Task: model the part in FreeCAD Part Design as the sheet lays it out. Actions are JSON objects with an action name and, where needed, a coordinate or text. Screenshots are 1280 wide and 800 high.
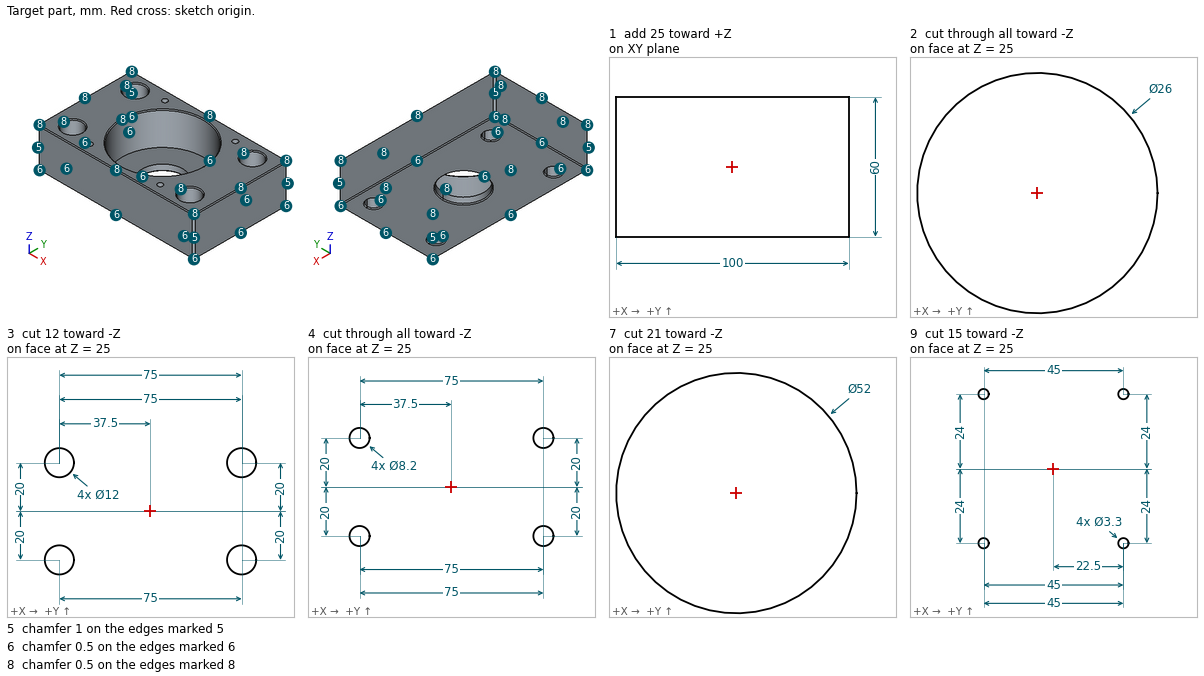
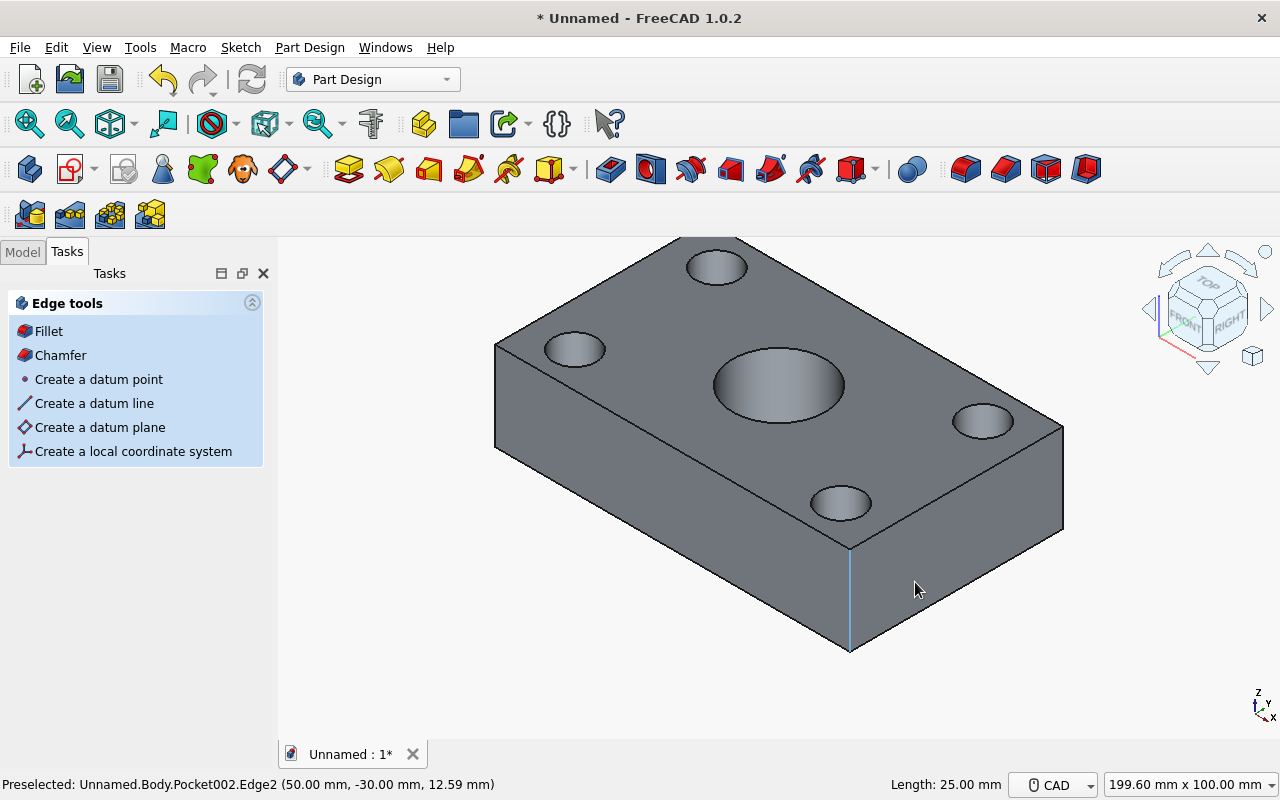
{"action": "key", "text": "v f"}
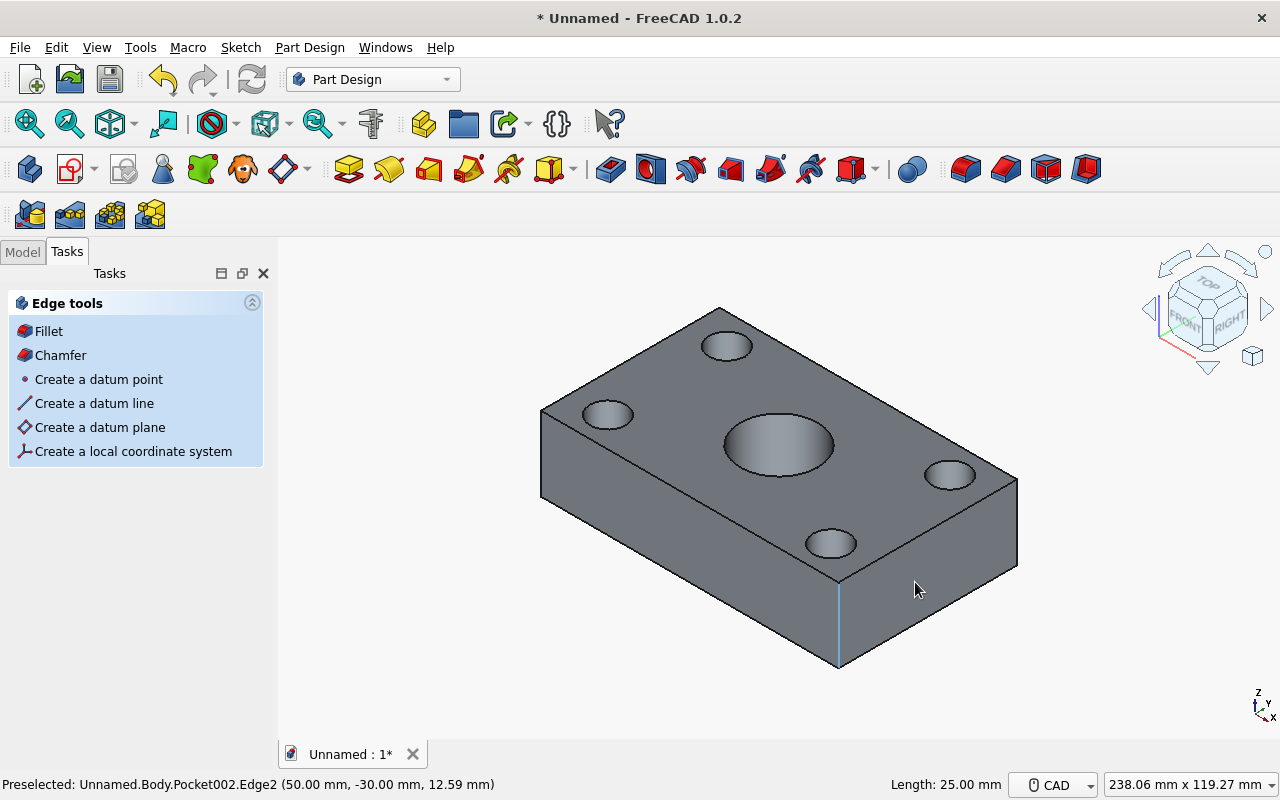
{"action": "key", "text": "2"}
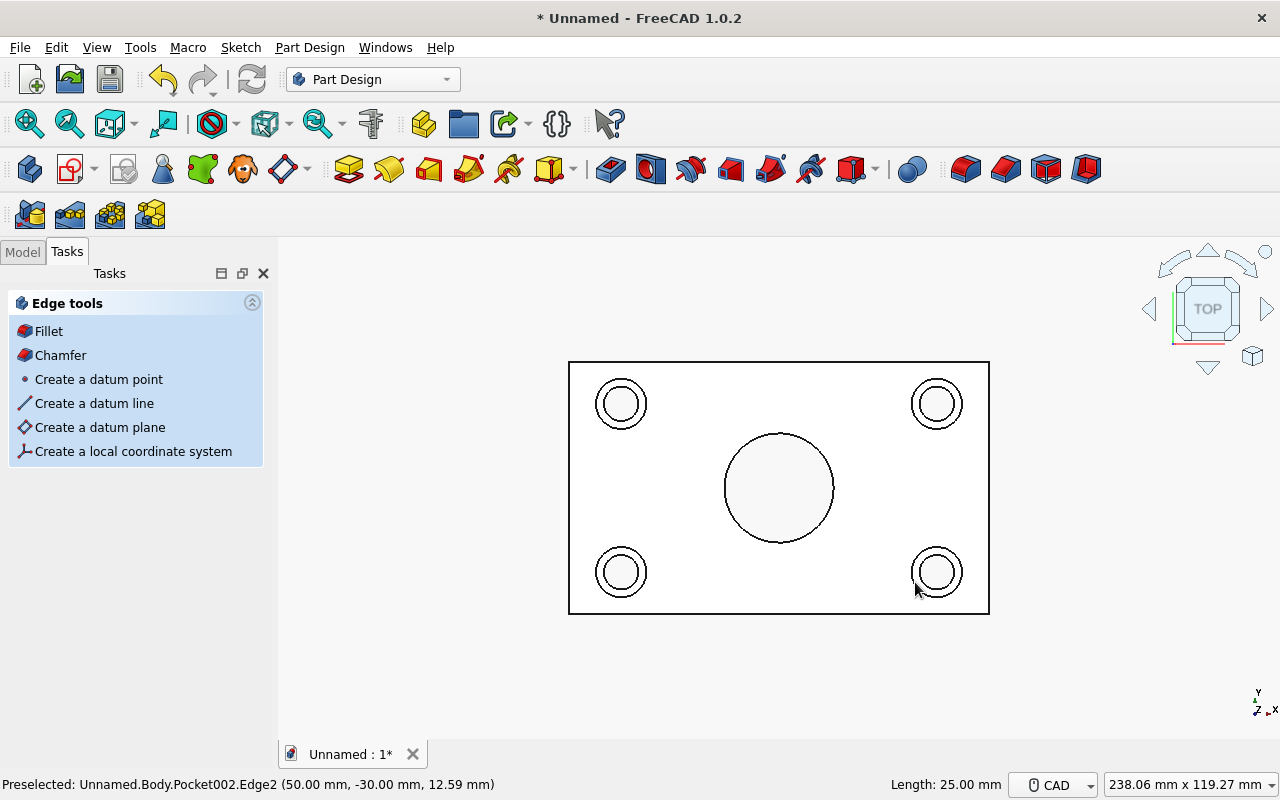
{"action": "key", "text": "1"}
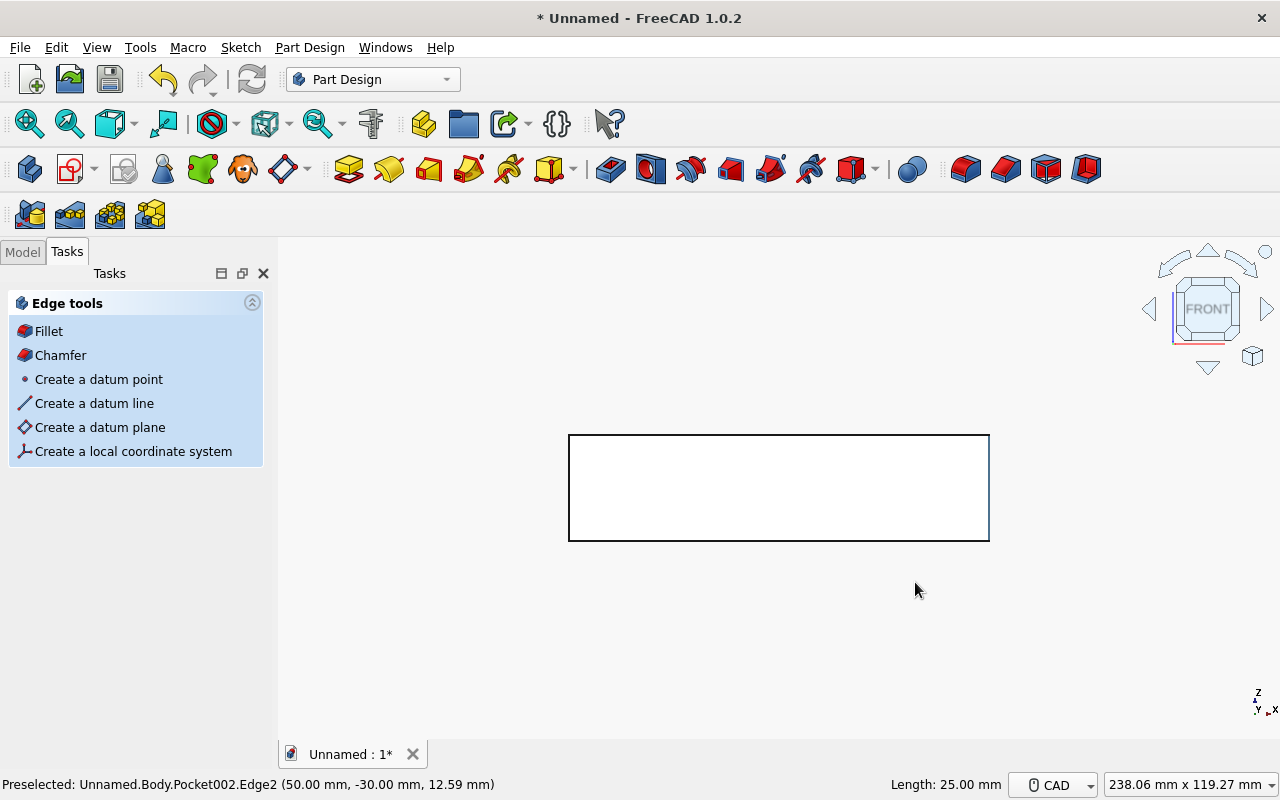
{"action": "left_click", "coordinate": [30, 124]}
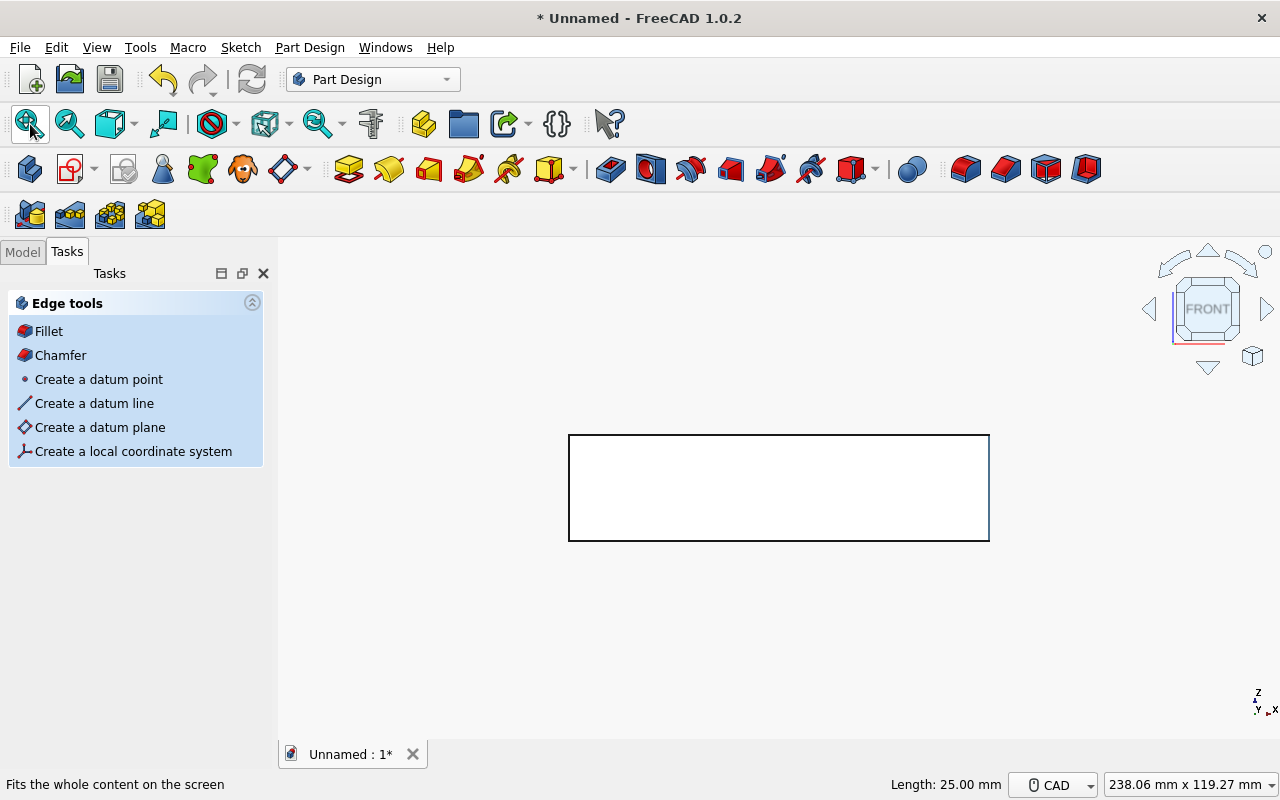
{"action": "left_click", "coordinate": [569, 487], "text": "ctrl"}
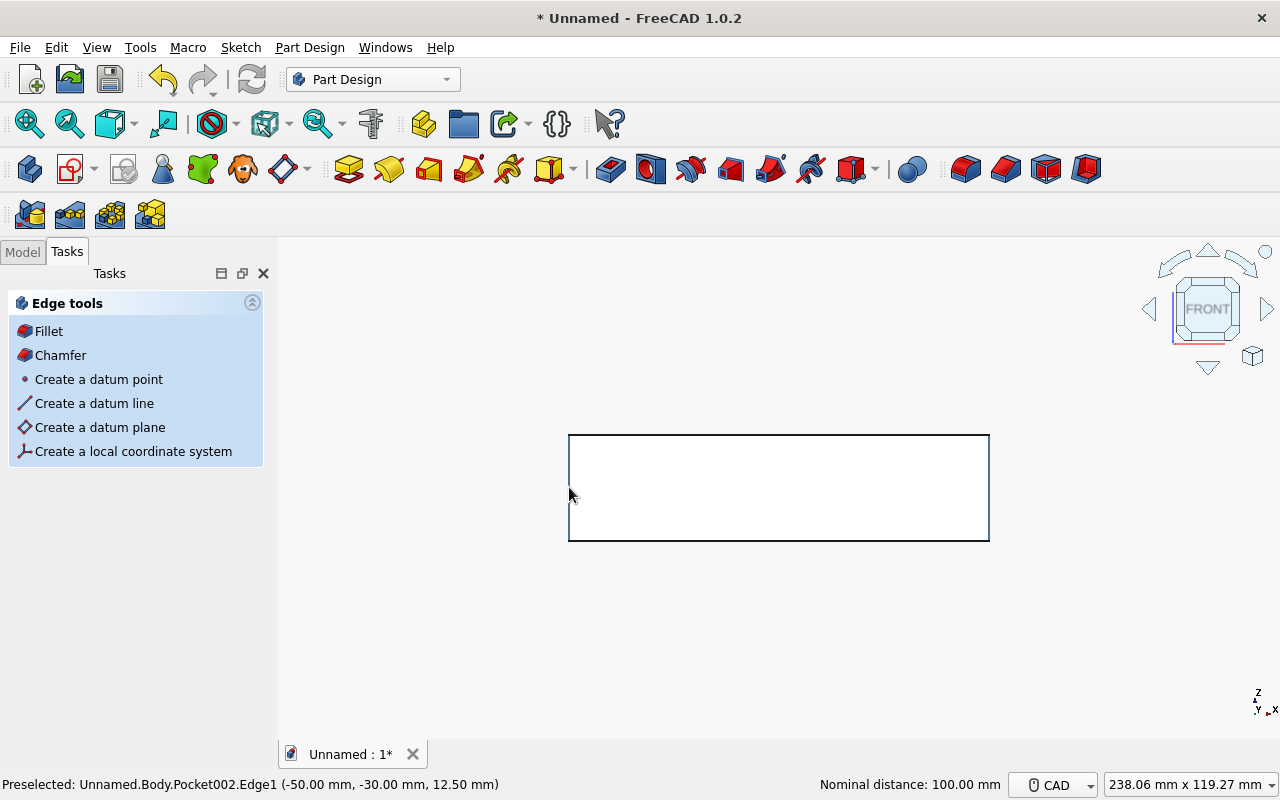
{"action": "key", "text": "3"}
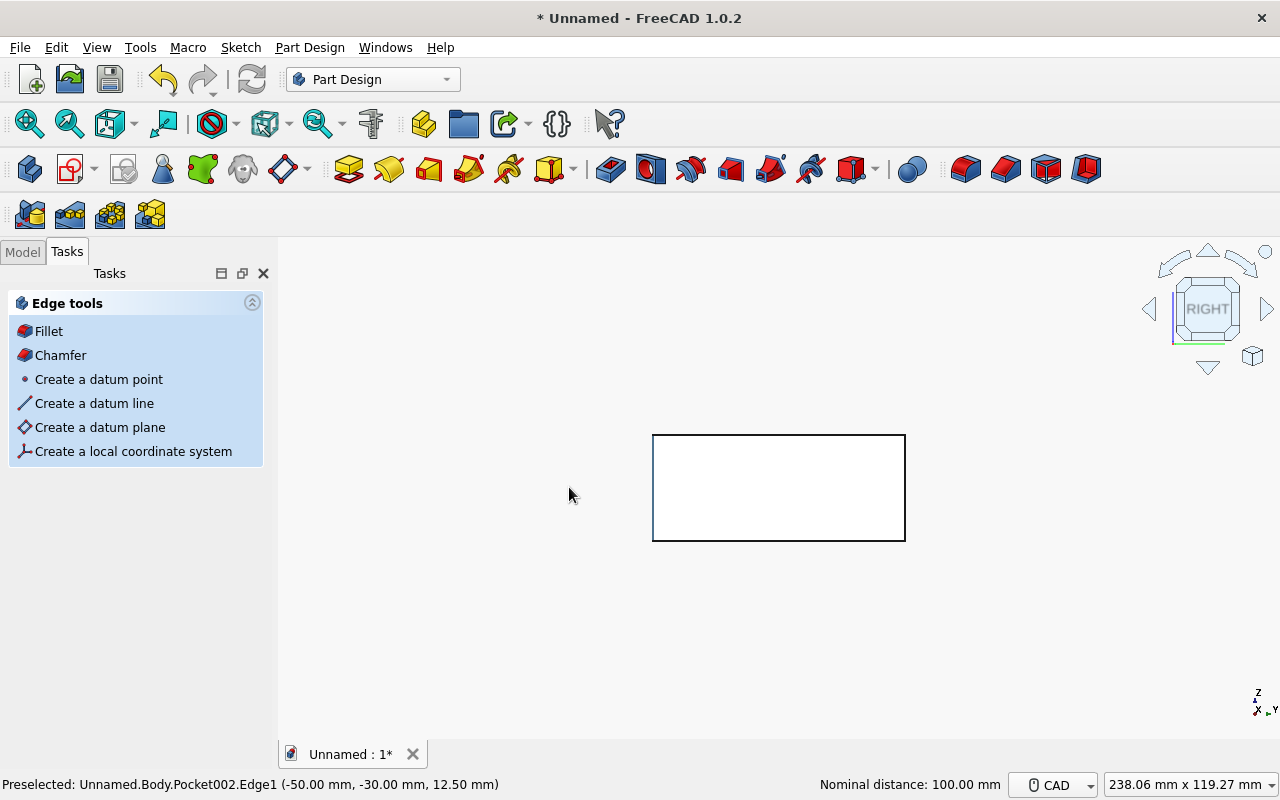
{"action": "left_click", "coordinate": [30, 124]}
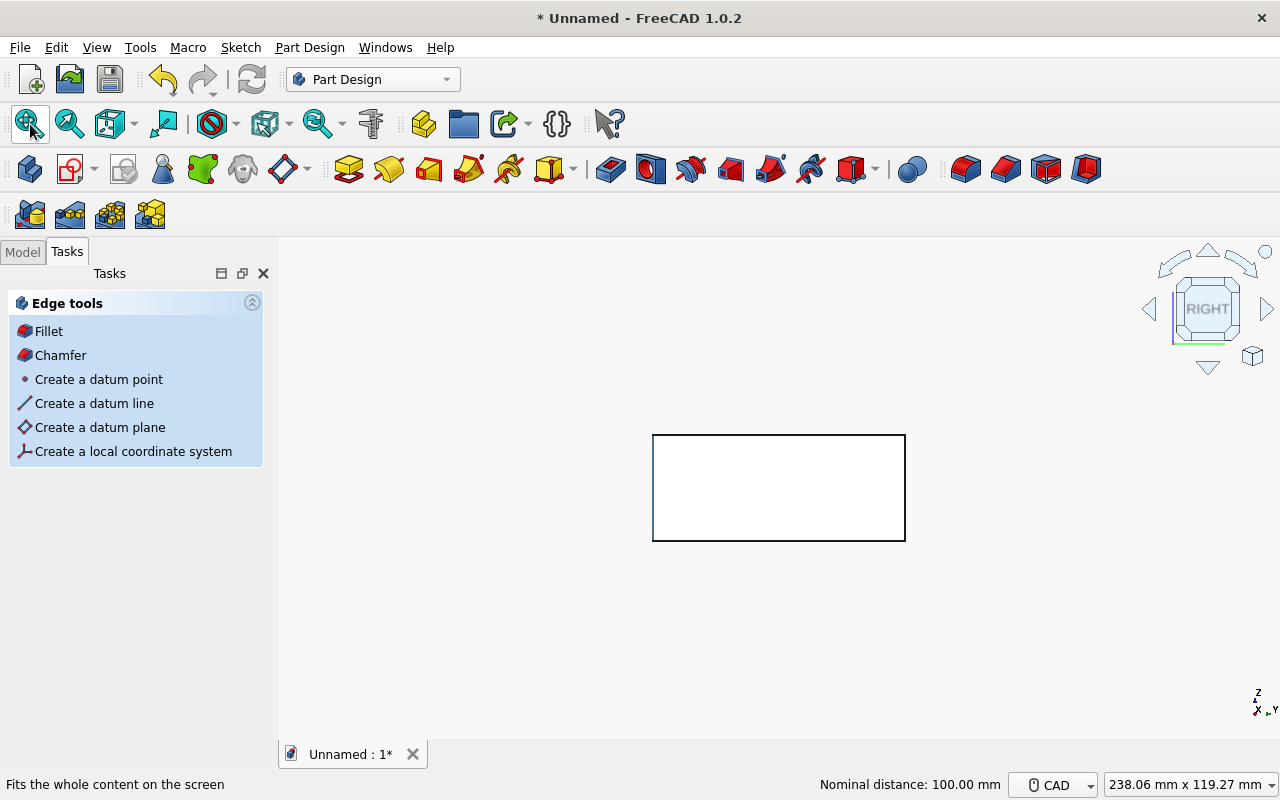
{"action": "left_click", "coordinate": [905, 487], "text": "ctrl"}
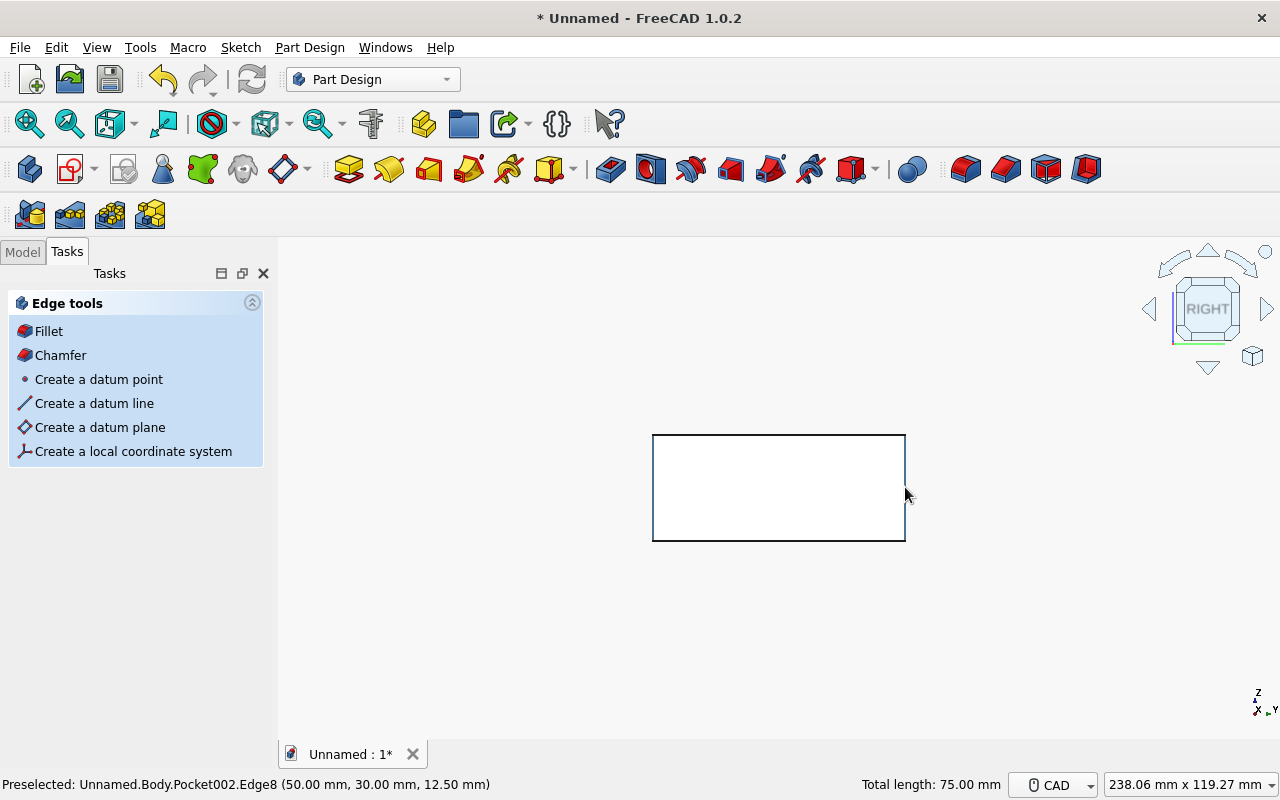
{"action": "key", "text": "5"}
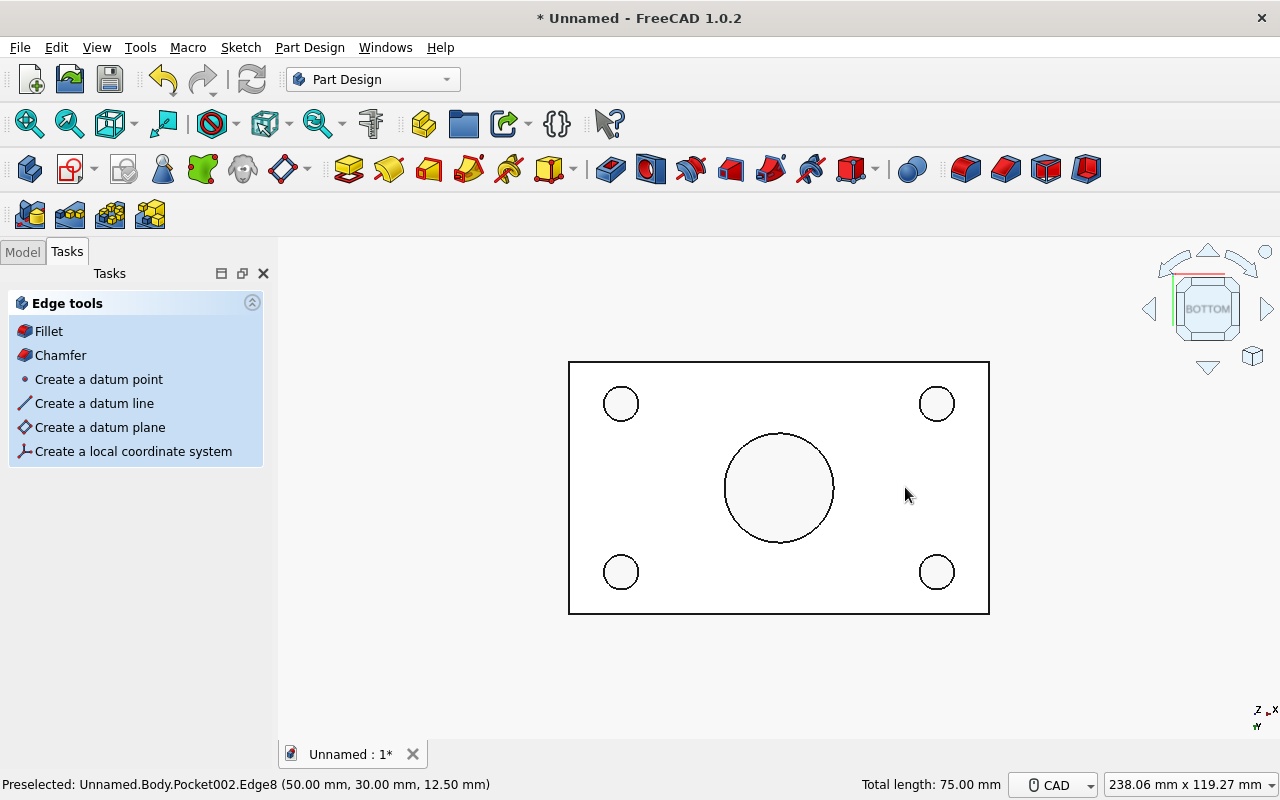
{"action": "key", "text": "4"}